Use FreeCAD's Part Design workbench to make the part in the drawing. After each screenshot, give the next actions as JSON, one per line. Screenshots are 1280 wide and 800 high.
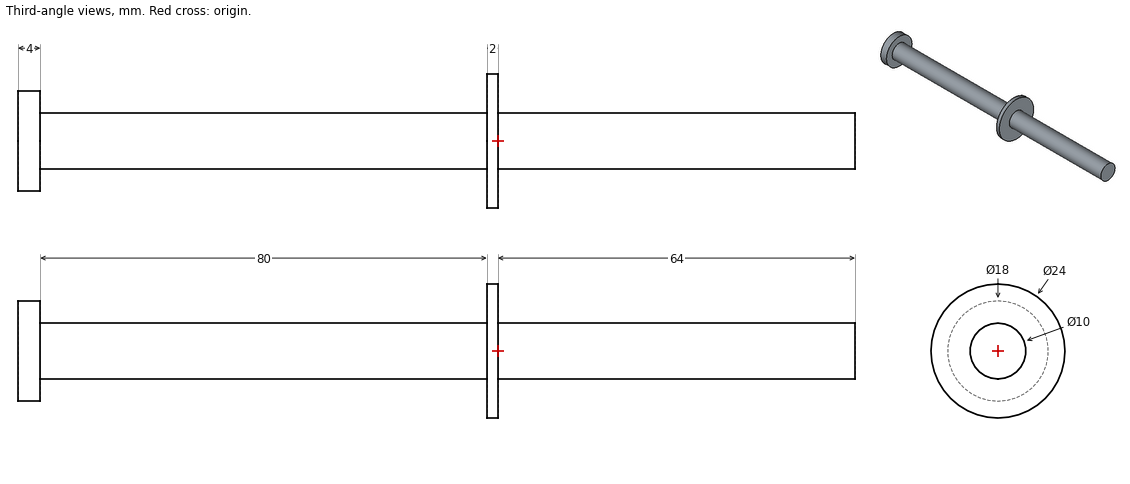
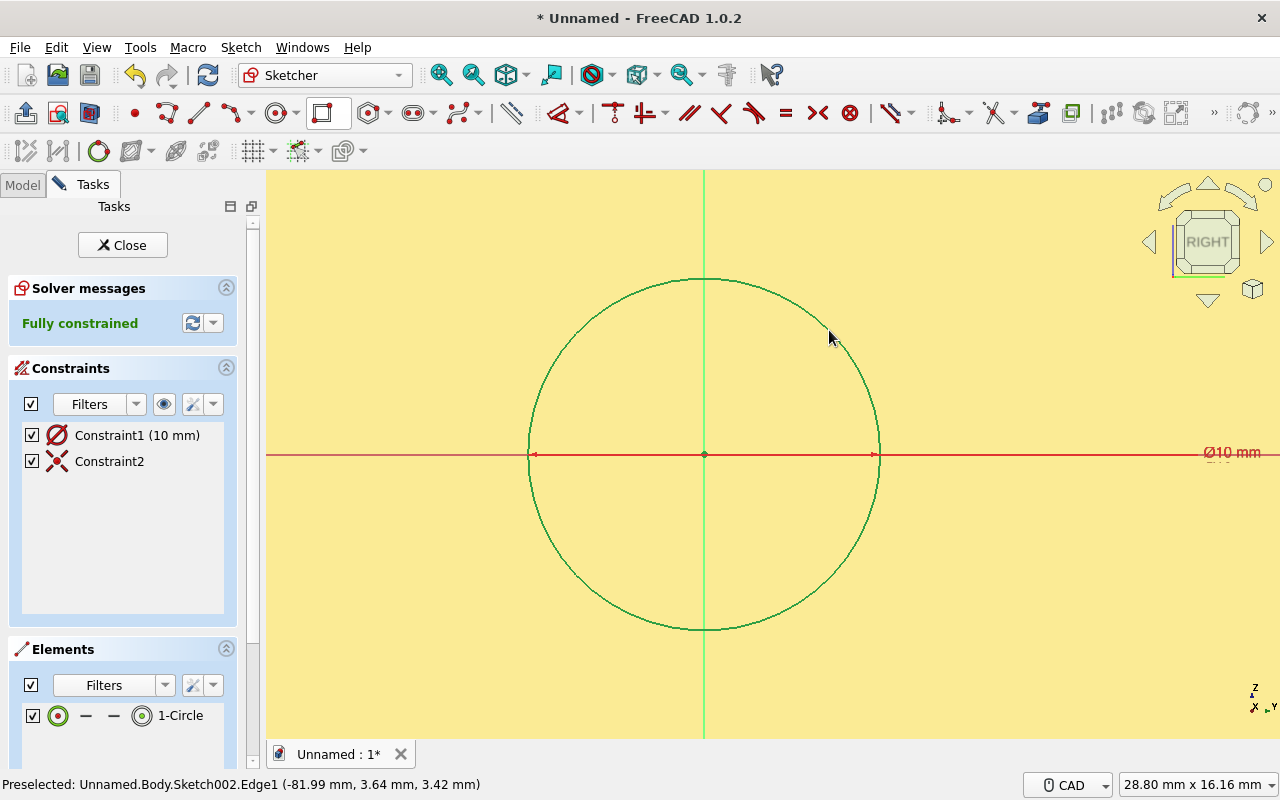
{"action": "left_click", "coordinate": [123, 245]}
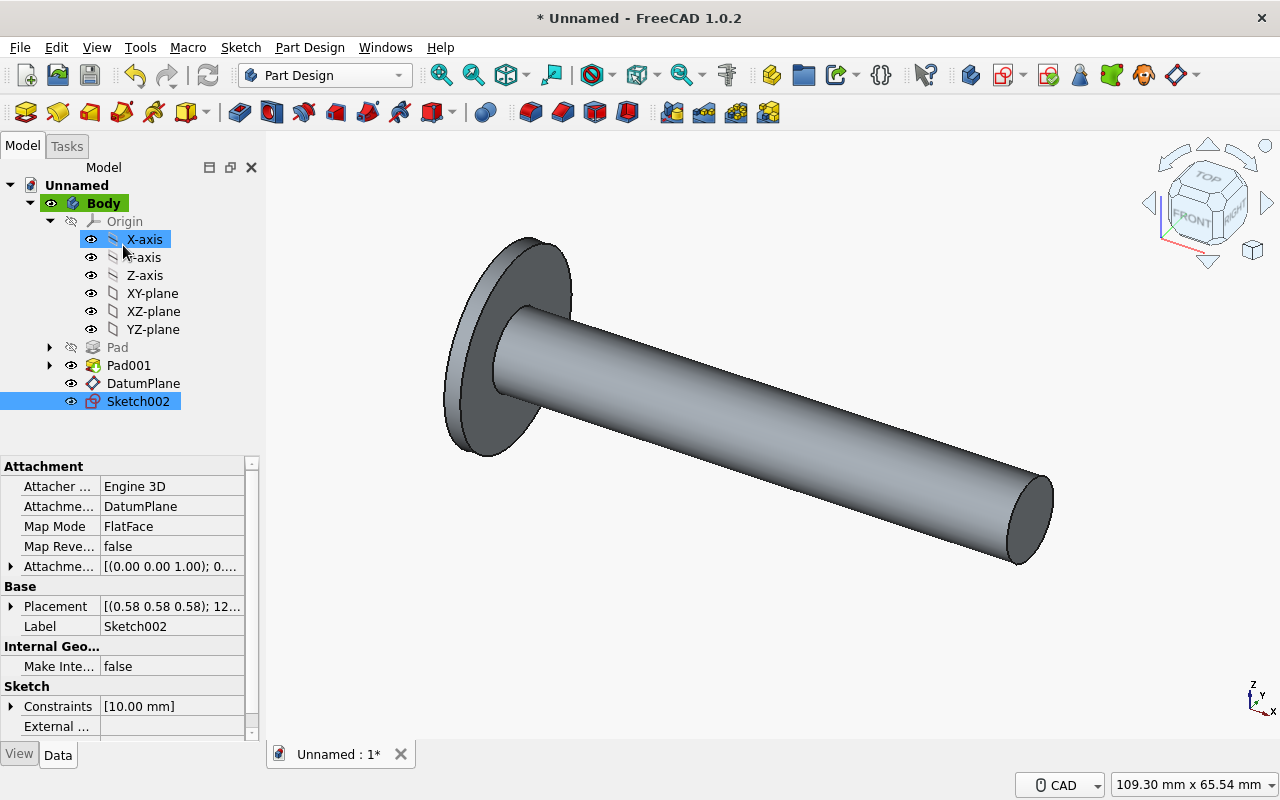
{"action": "left_click", "coordinate": [26, 112]}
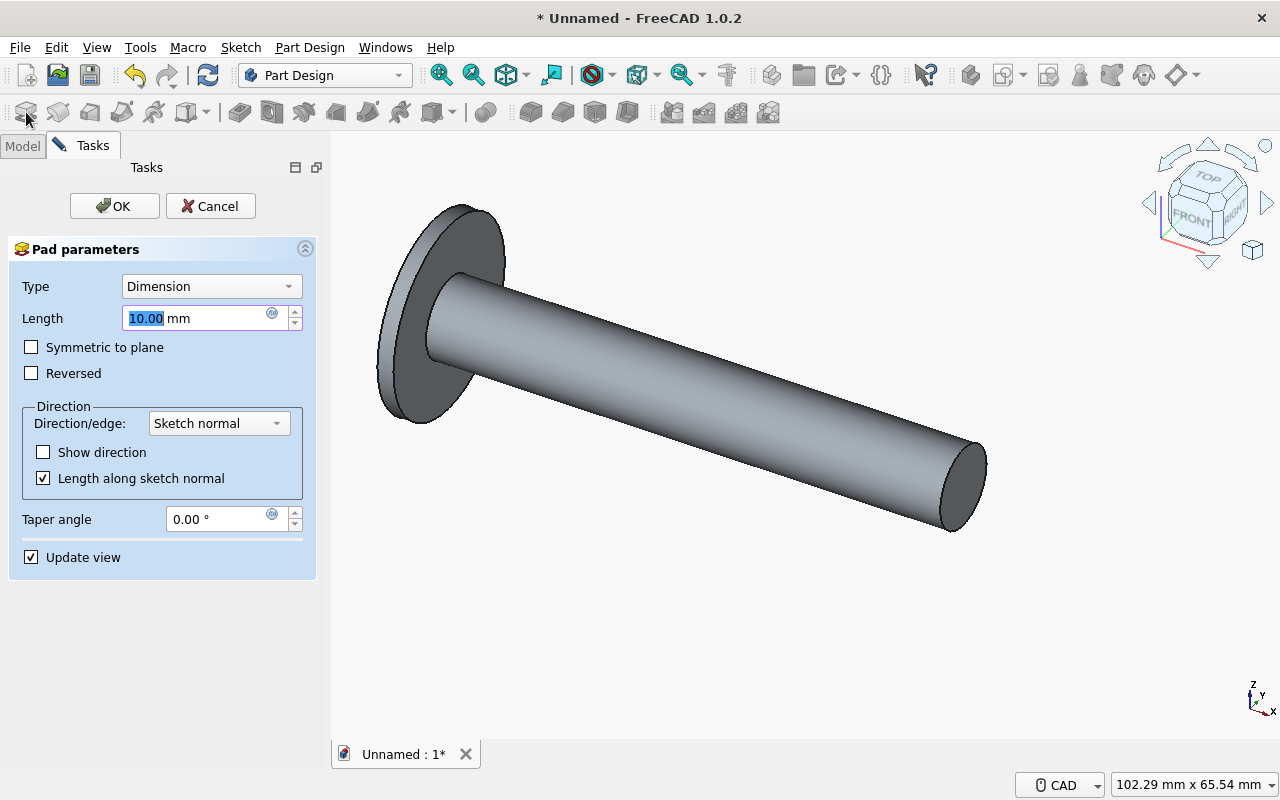
{"action": "type", "text": "80"}
{"action": "key", "text": "Tab"}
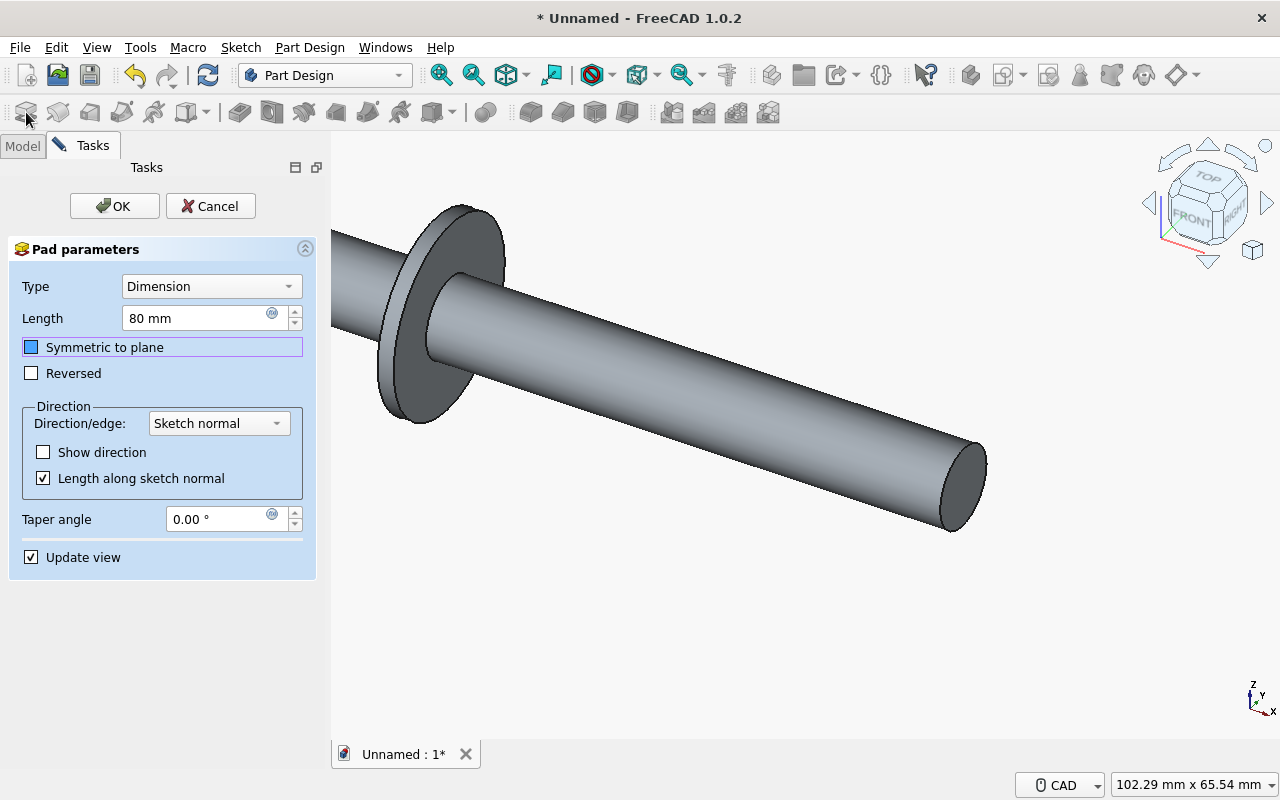
{"action": "left_click", "coordinate": [115, 206]}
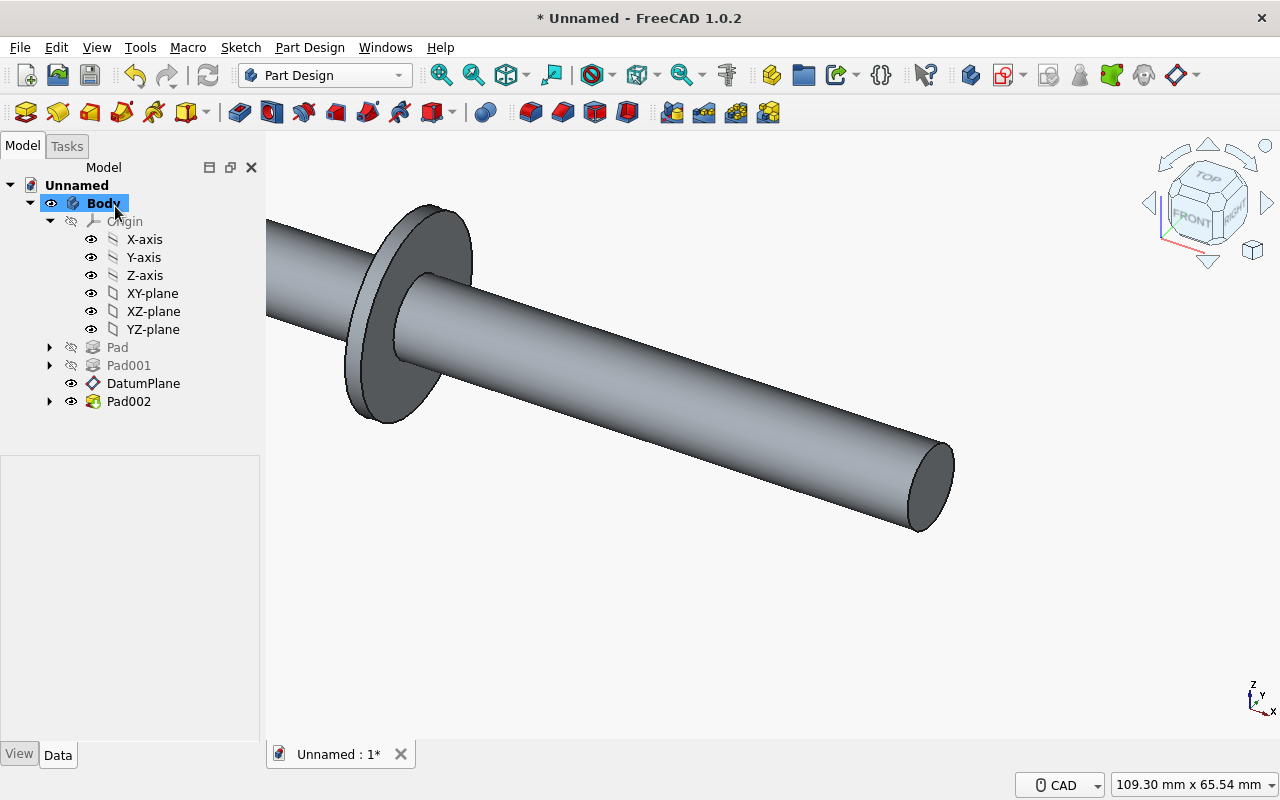
{"action": "left_click", "coordinate": [116, 383]}
{"action": "key", "text": "space"}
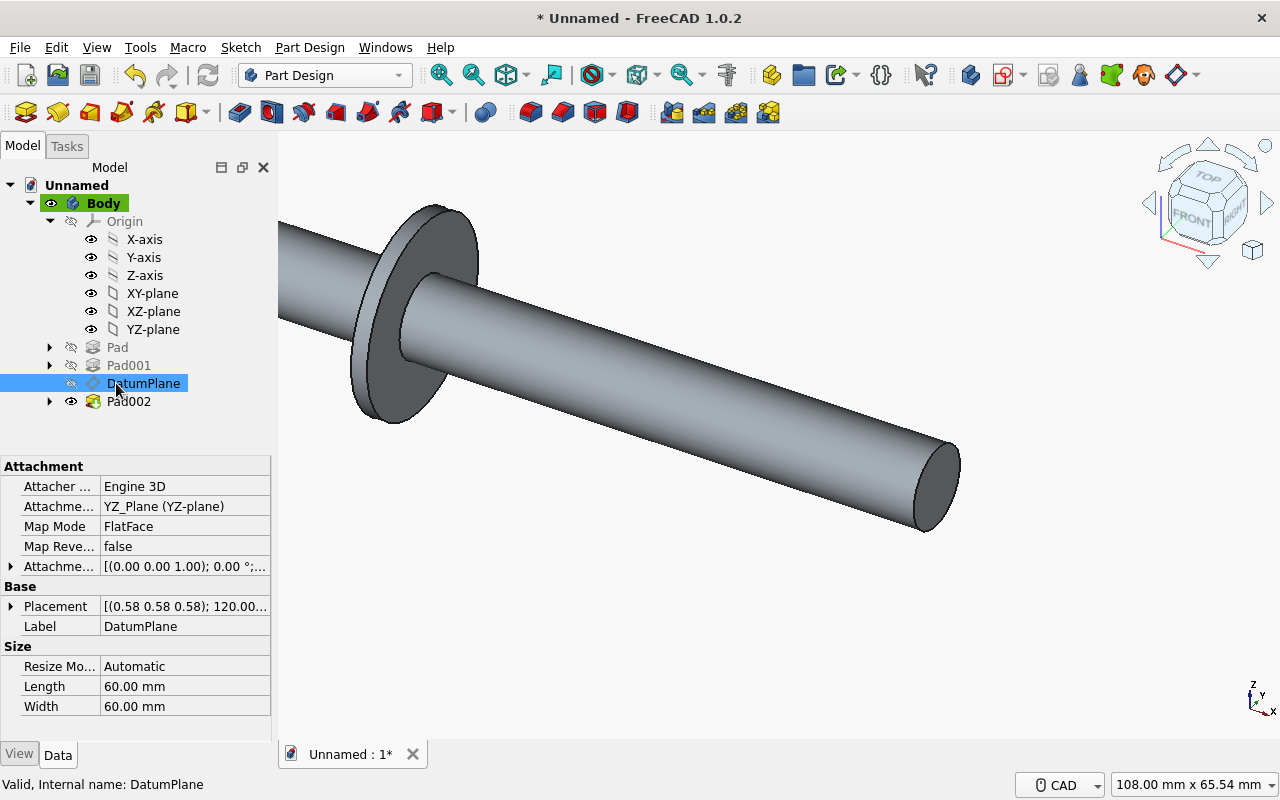
{"action": "key", "text": "v f"}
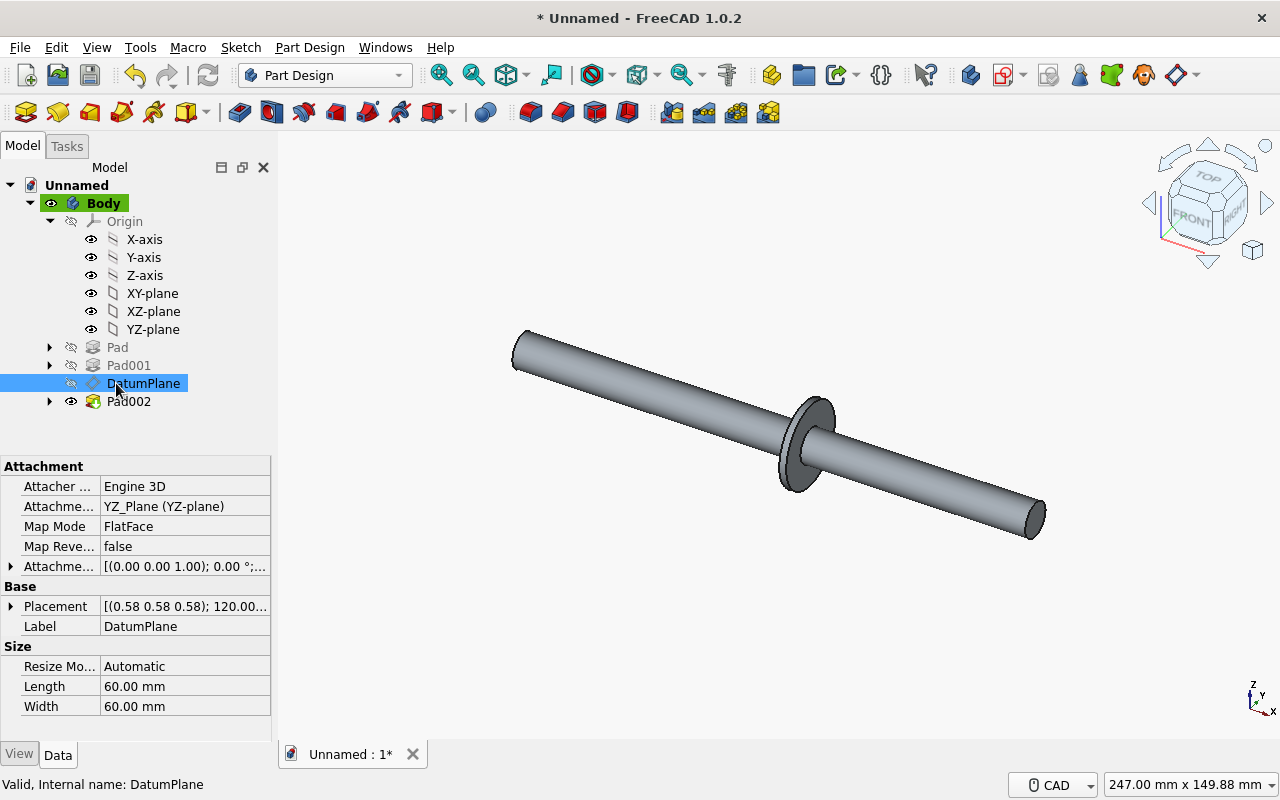
{"action": "key", "text": "6"}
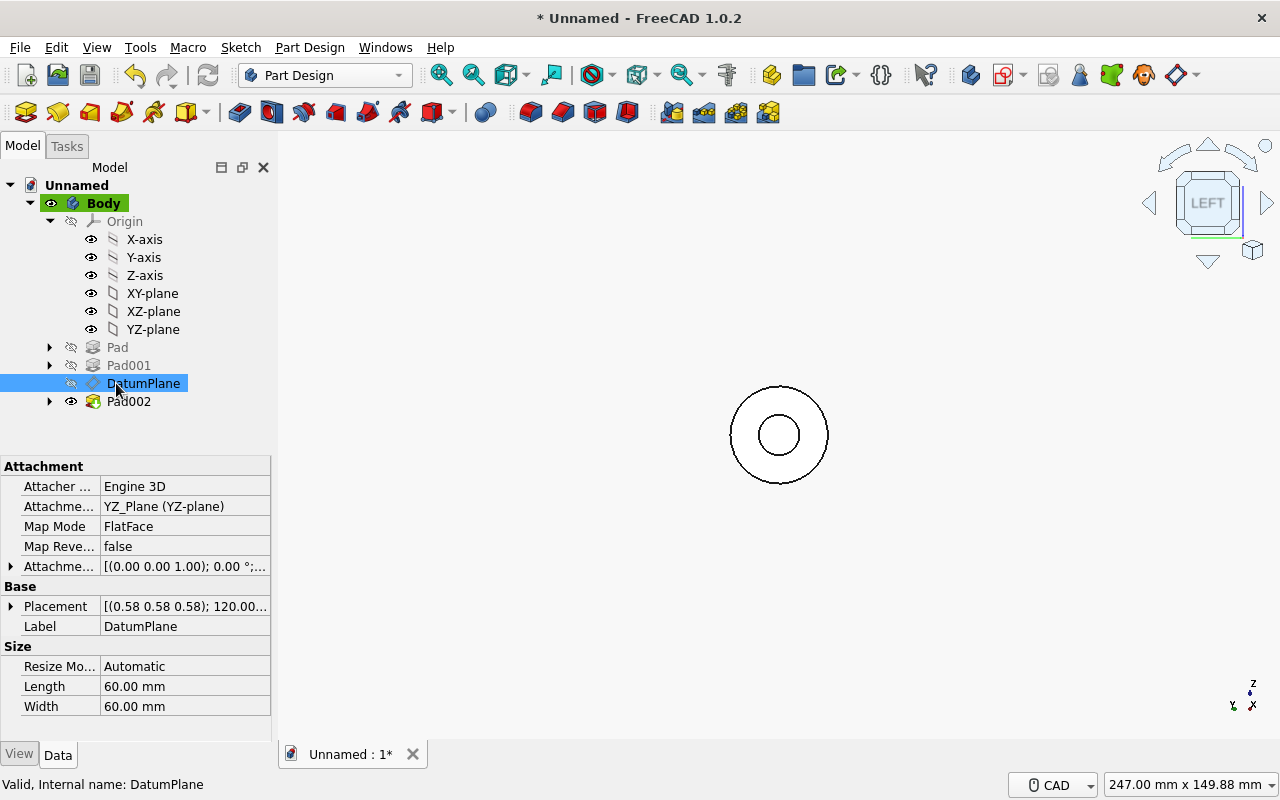
{"action": "key", "text": "v f"}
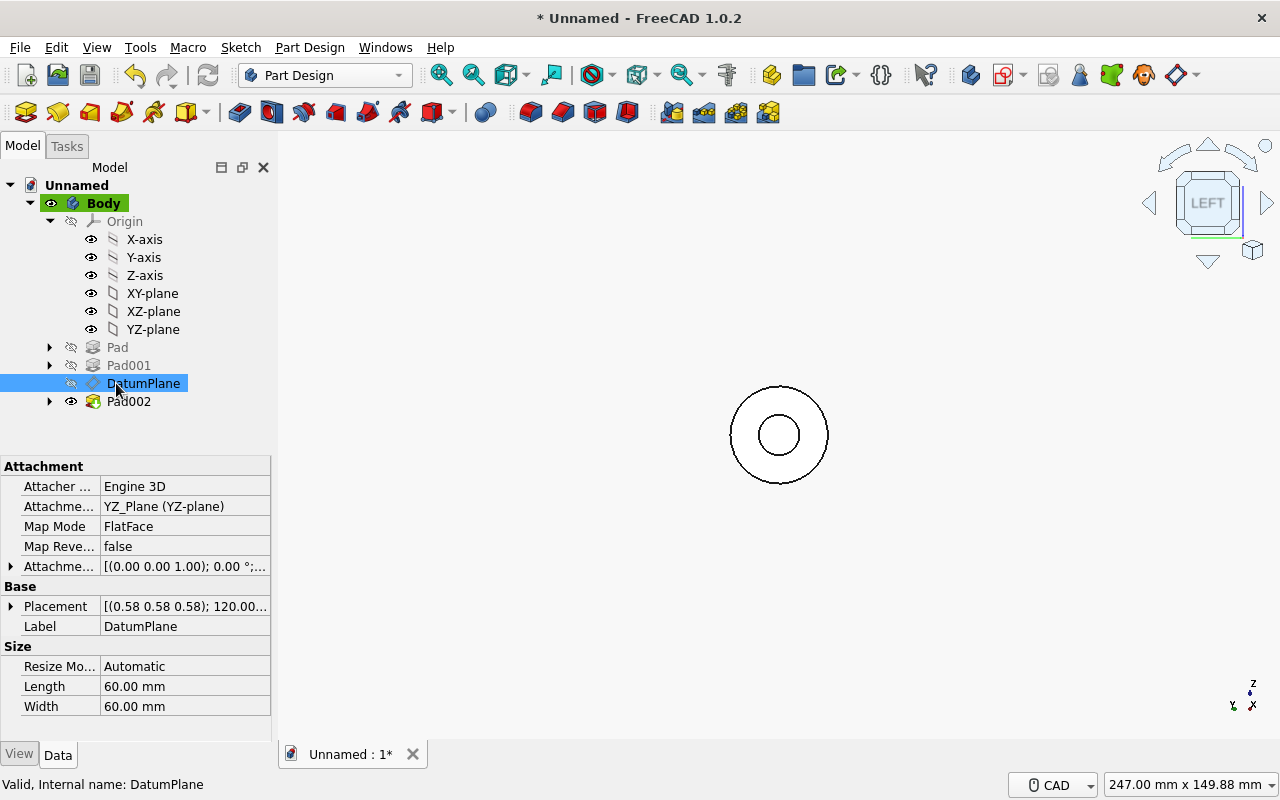
{"action": "left_click", "coordinate": [779, 434]}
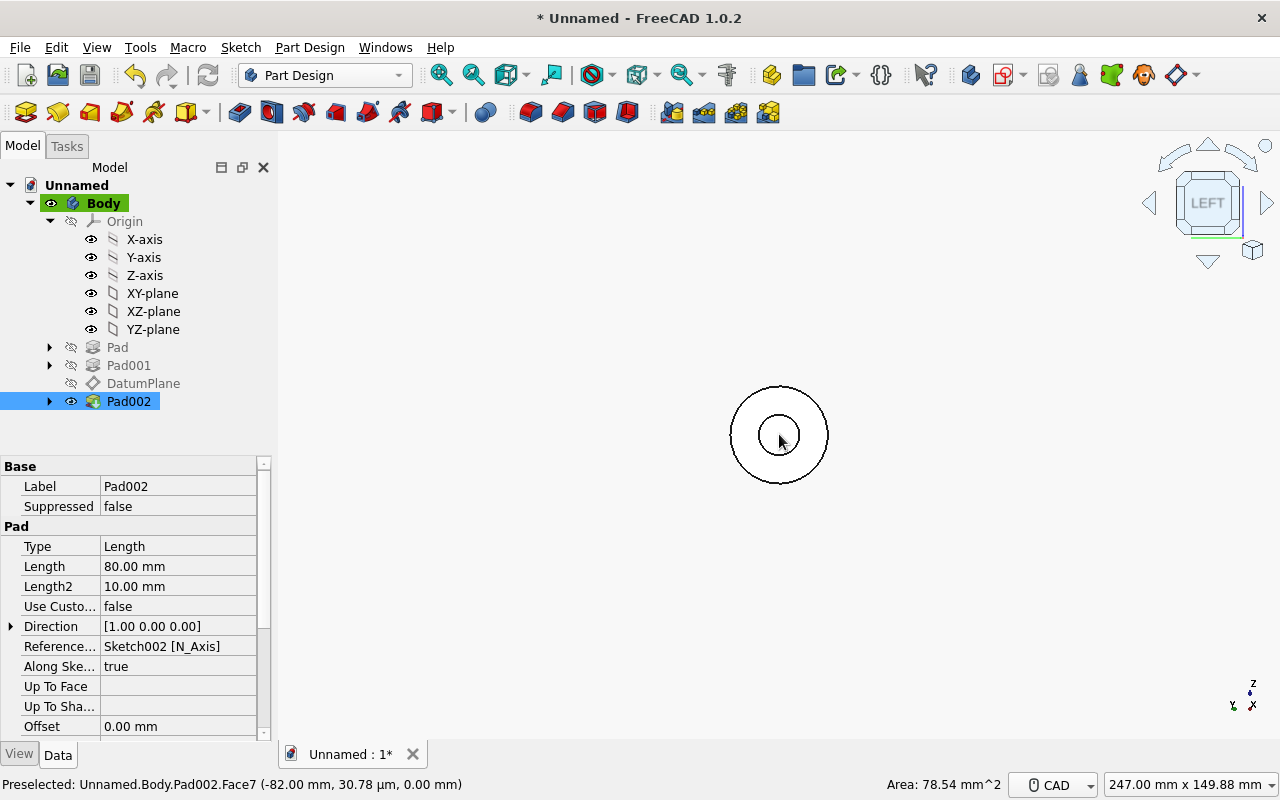
{"action": "left_click", "coordinate": [1004, 76]}